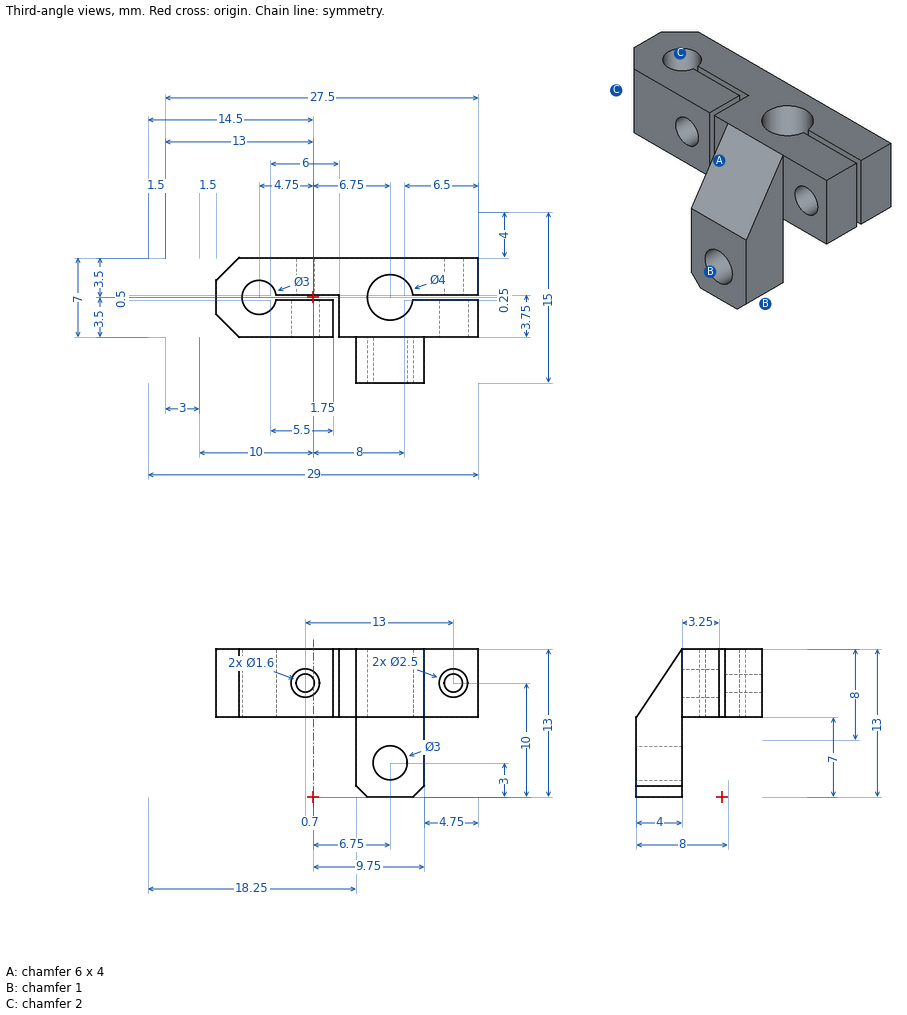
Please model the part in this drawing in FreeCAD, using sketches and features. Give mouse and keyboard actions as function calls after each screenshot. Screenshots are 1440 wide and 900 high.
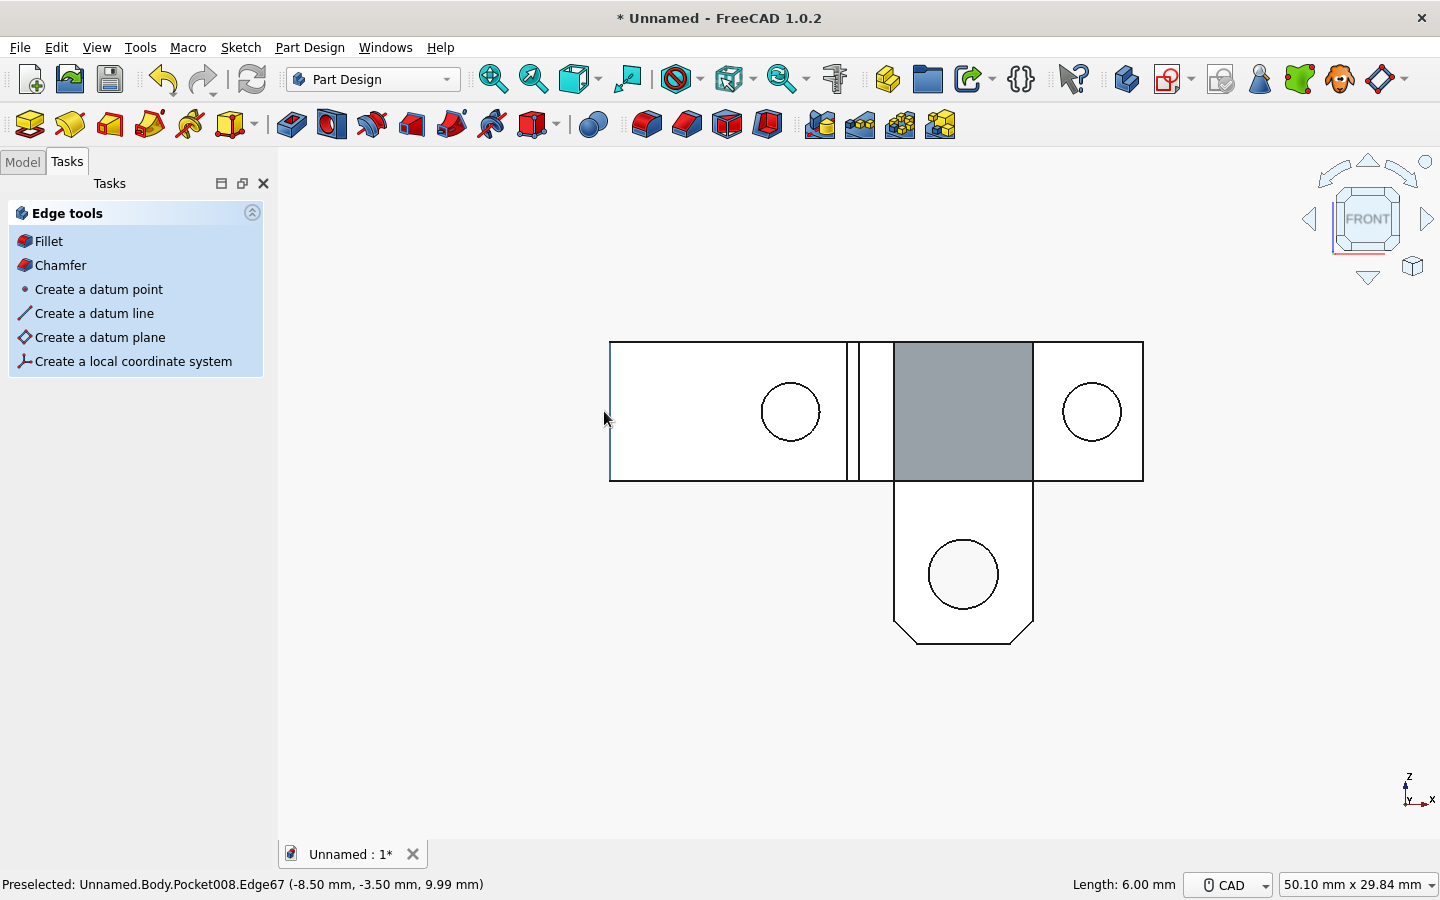
key(3)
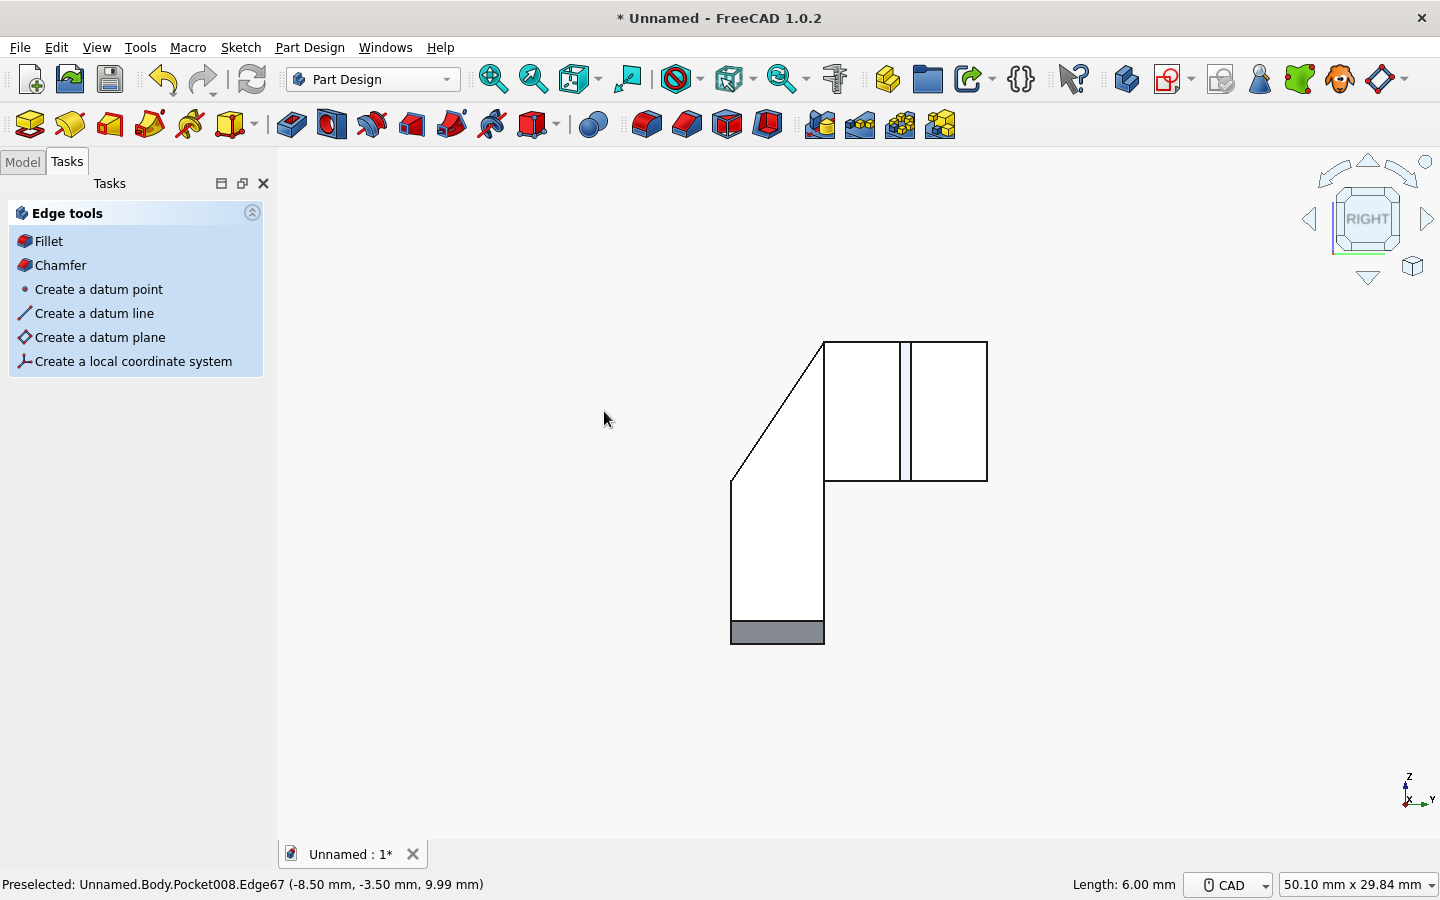
click(494, 80)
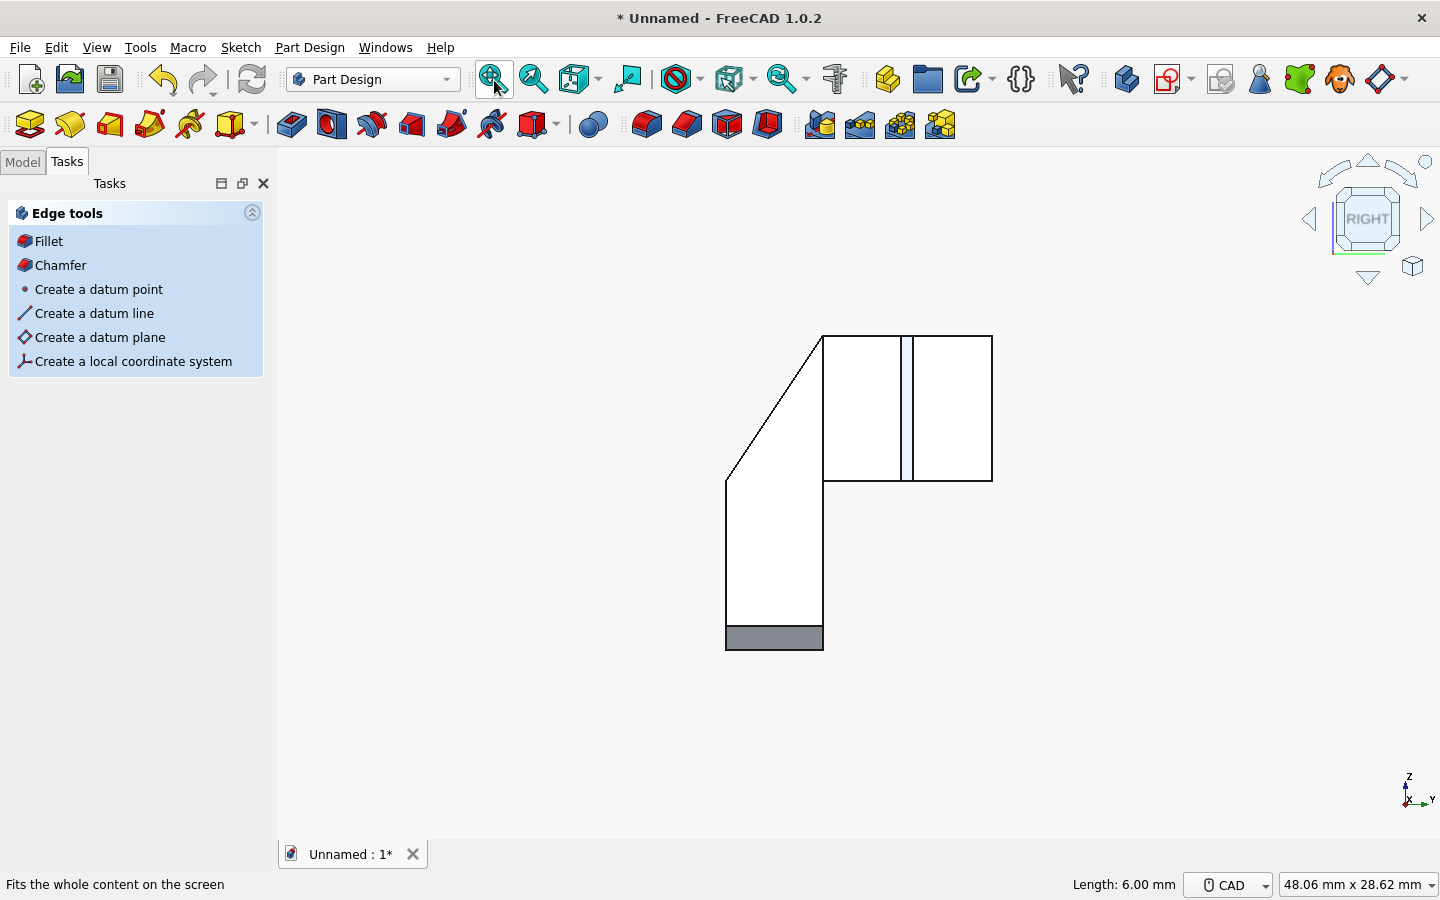
key(5)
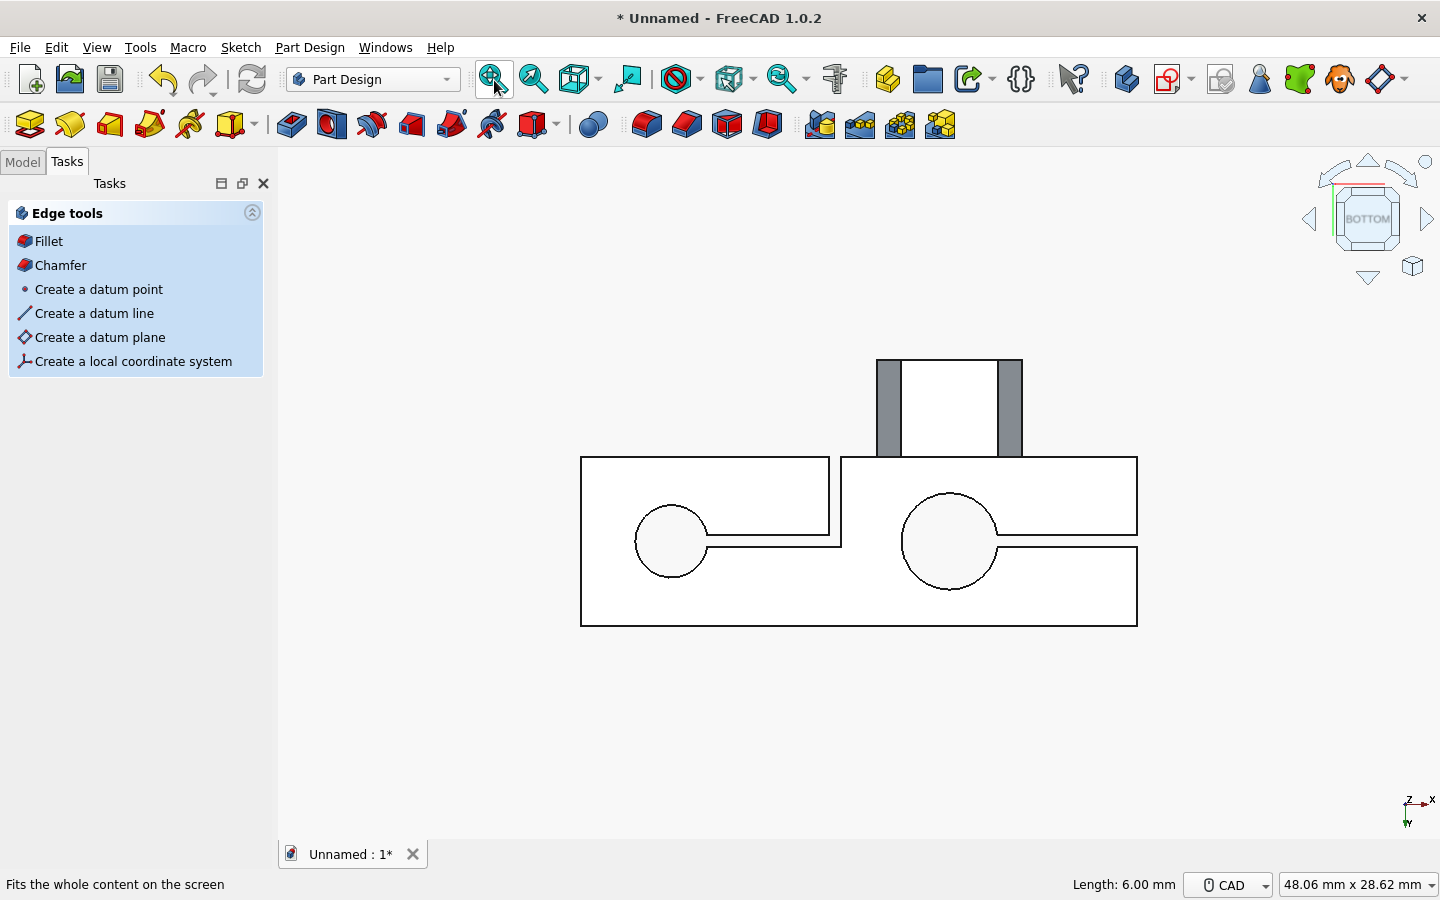
key(4)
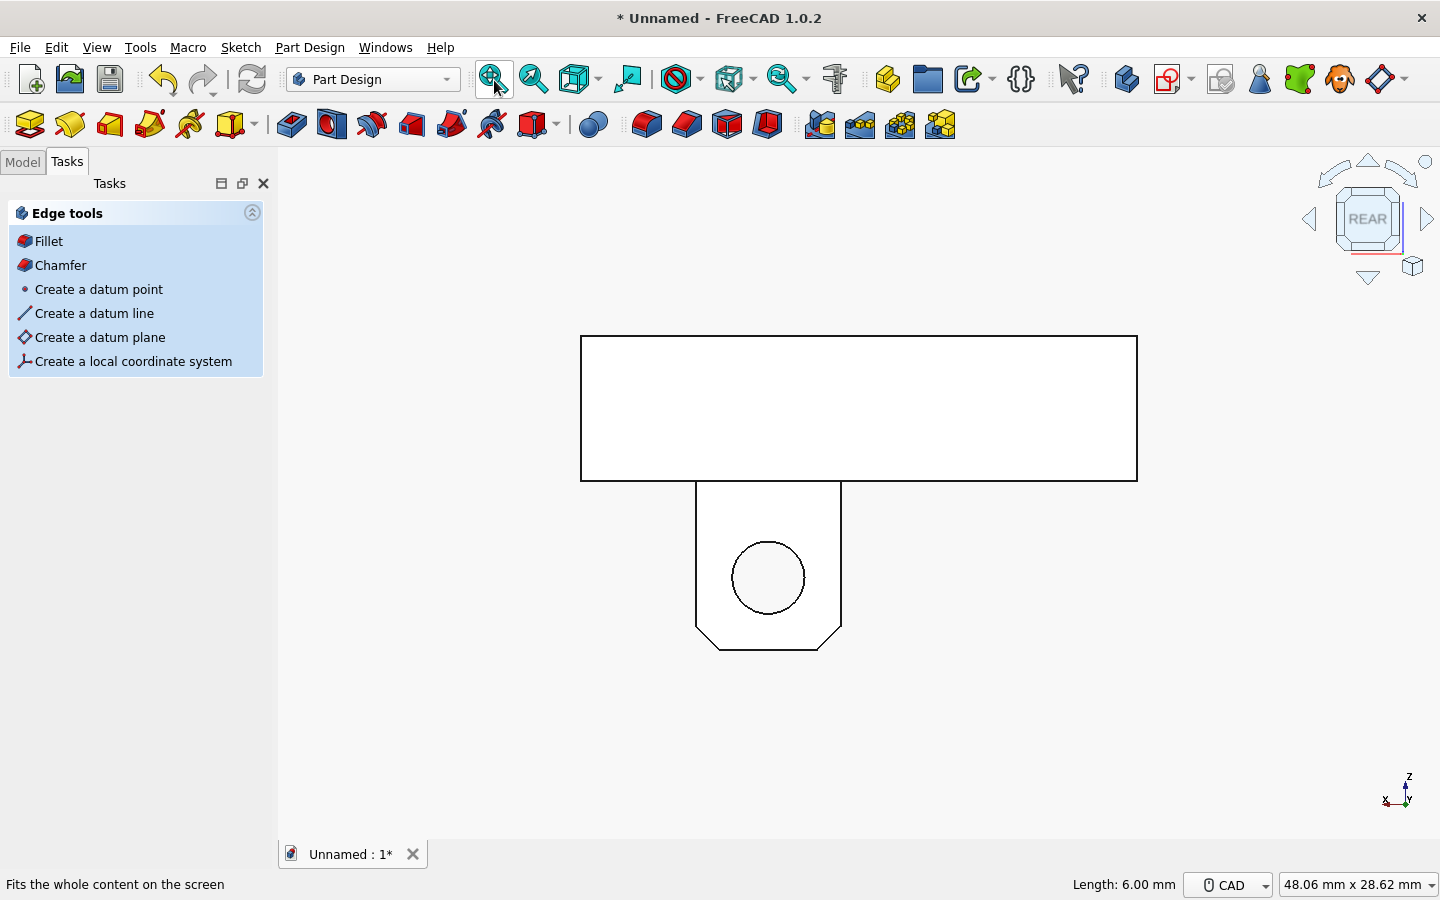
click(1137, 407, ctrl)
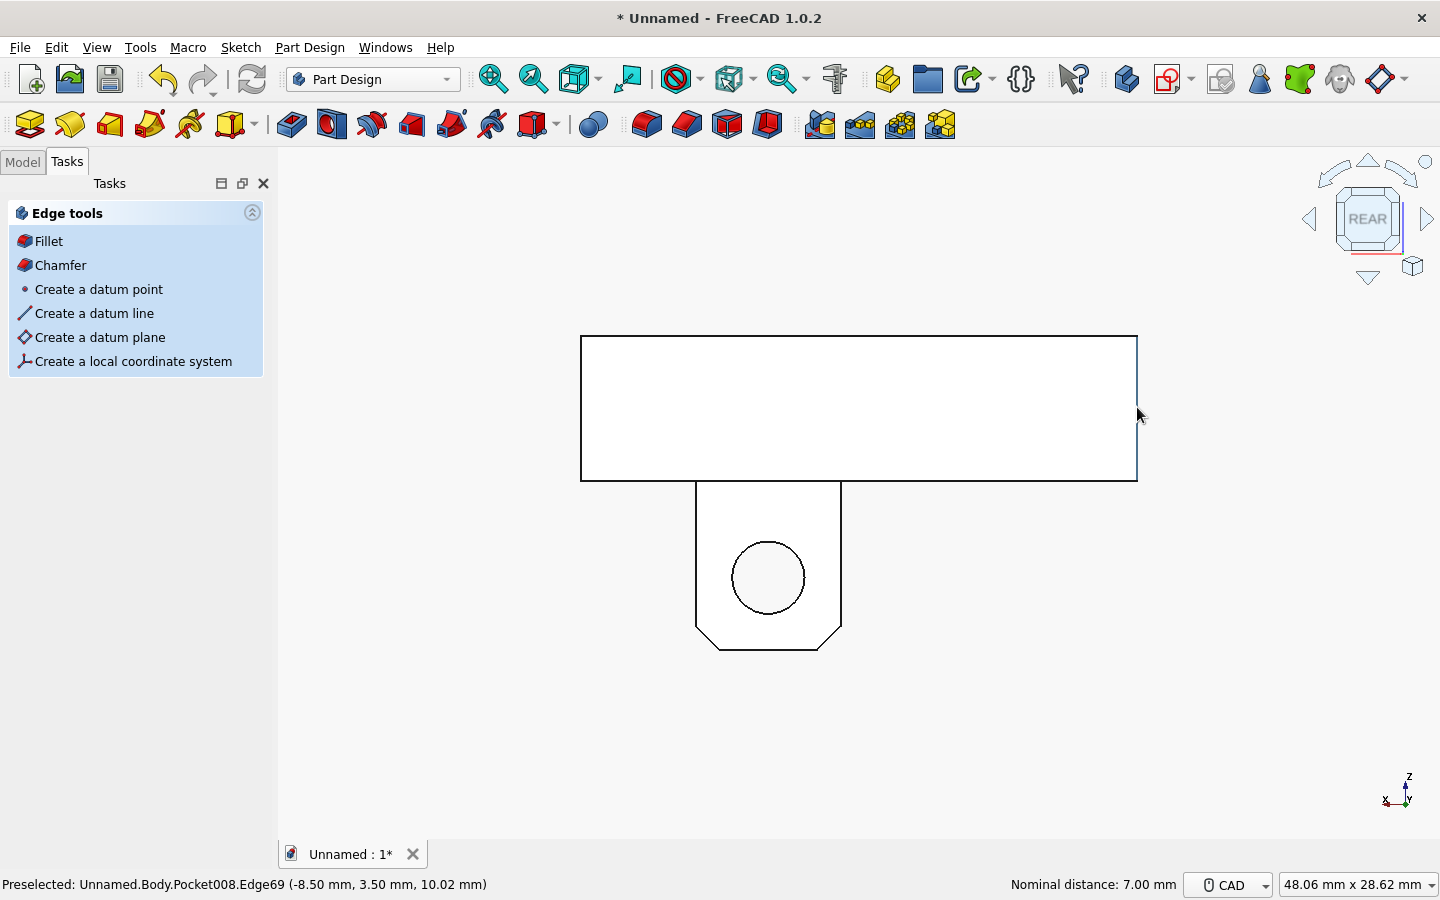
click(688, 124)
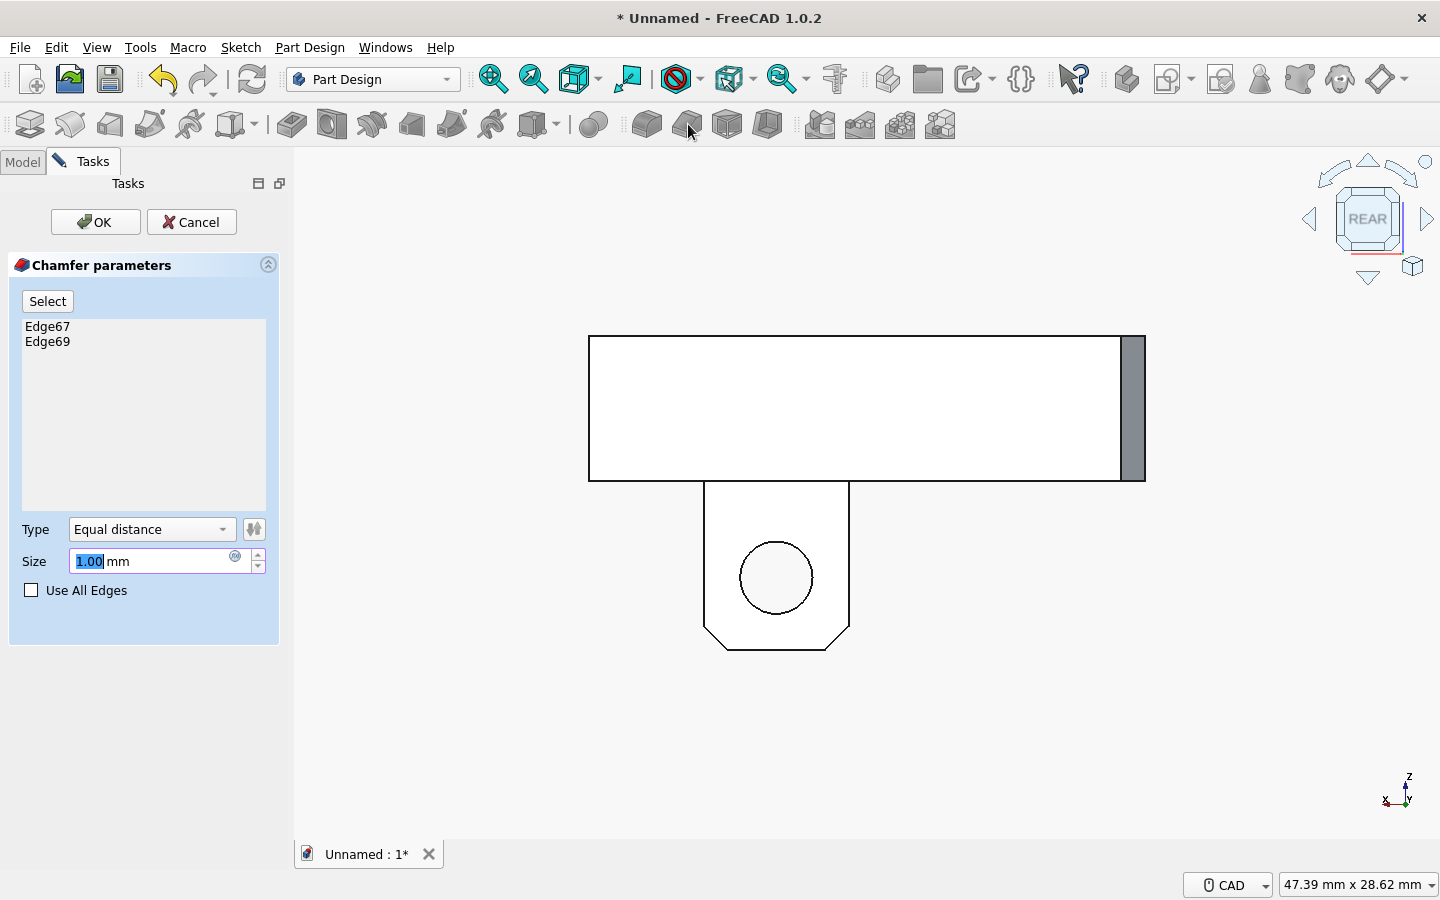
text(2)
key(Tab)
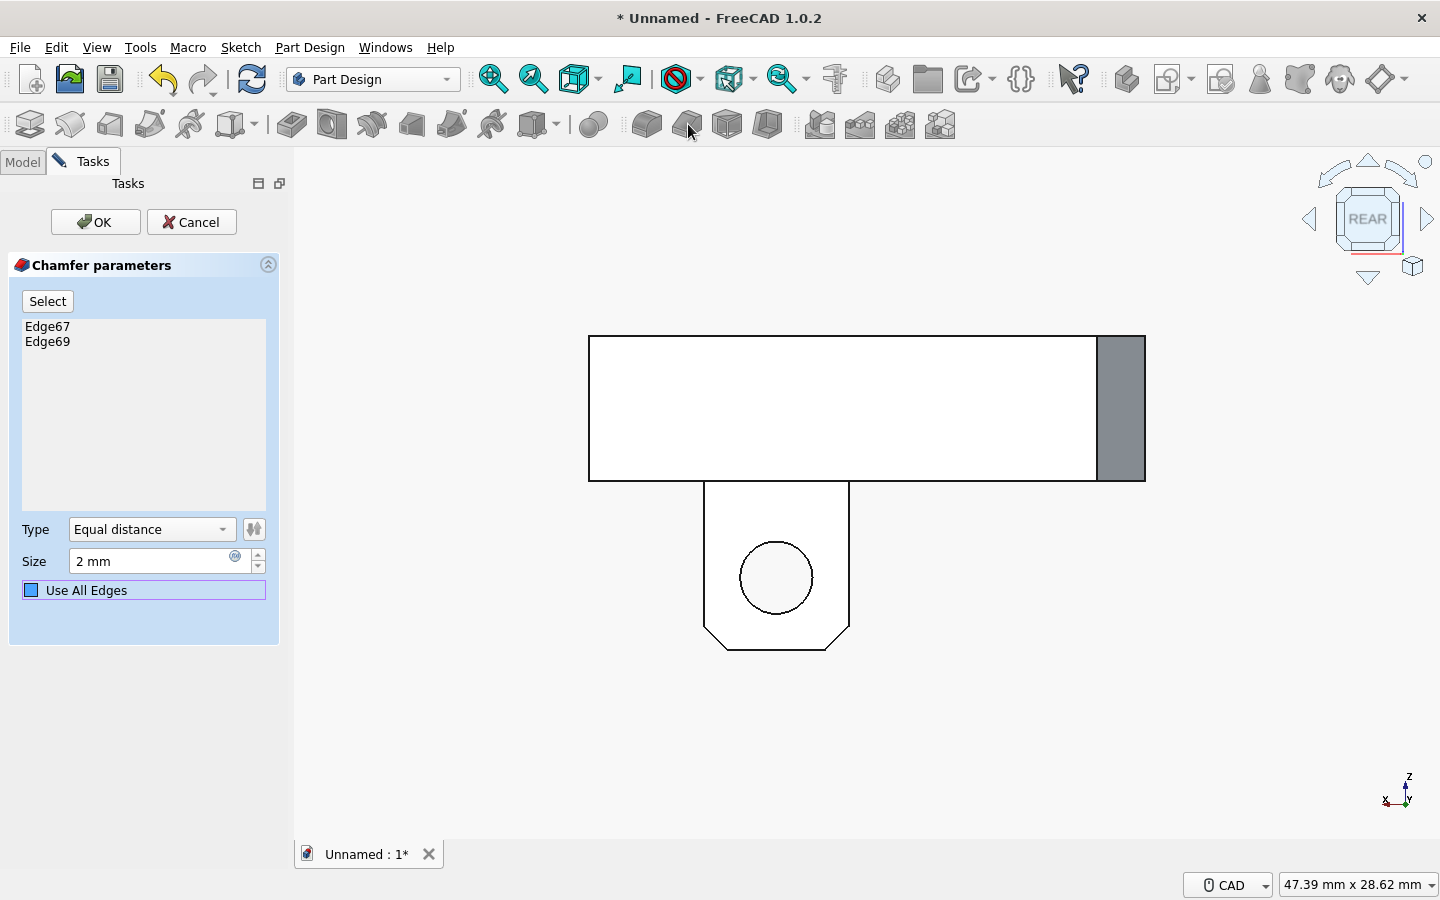
click(96, 222)